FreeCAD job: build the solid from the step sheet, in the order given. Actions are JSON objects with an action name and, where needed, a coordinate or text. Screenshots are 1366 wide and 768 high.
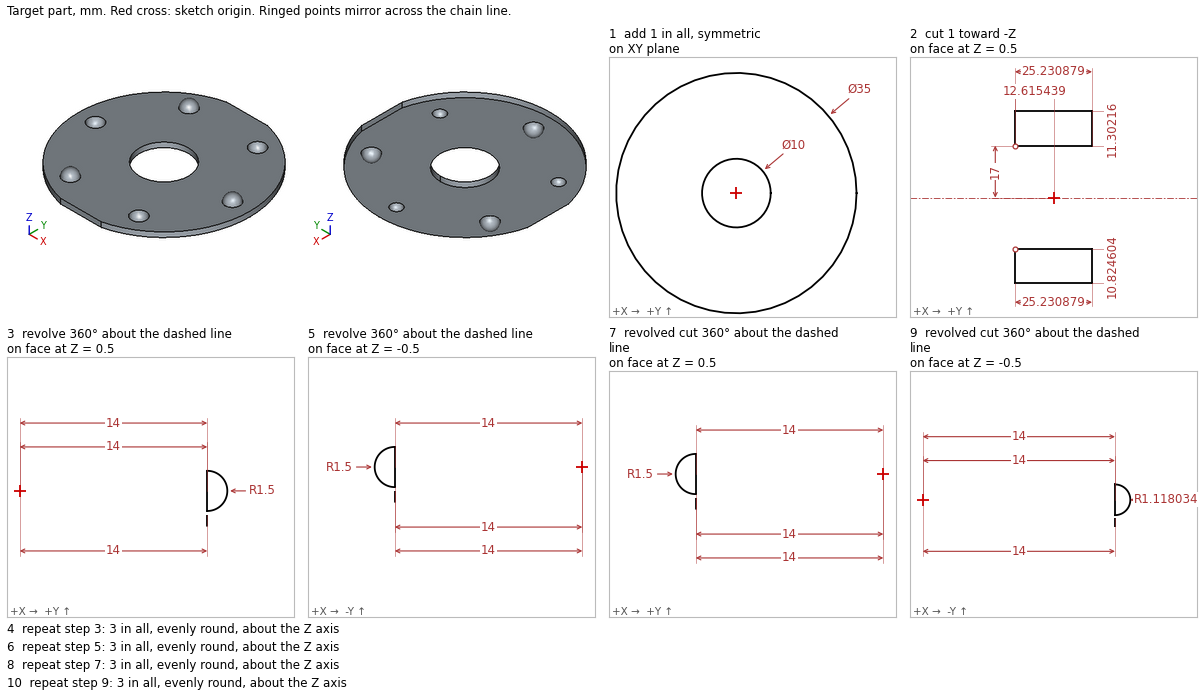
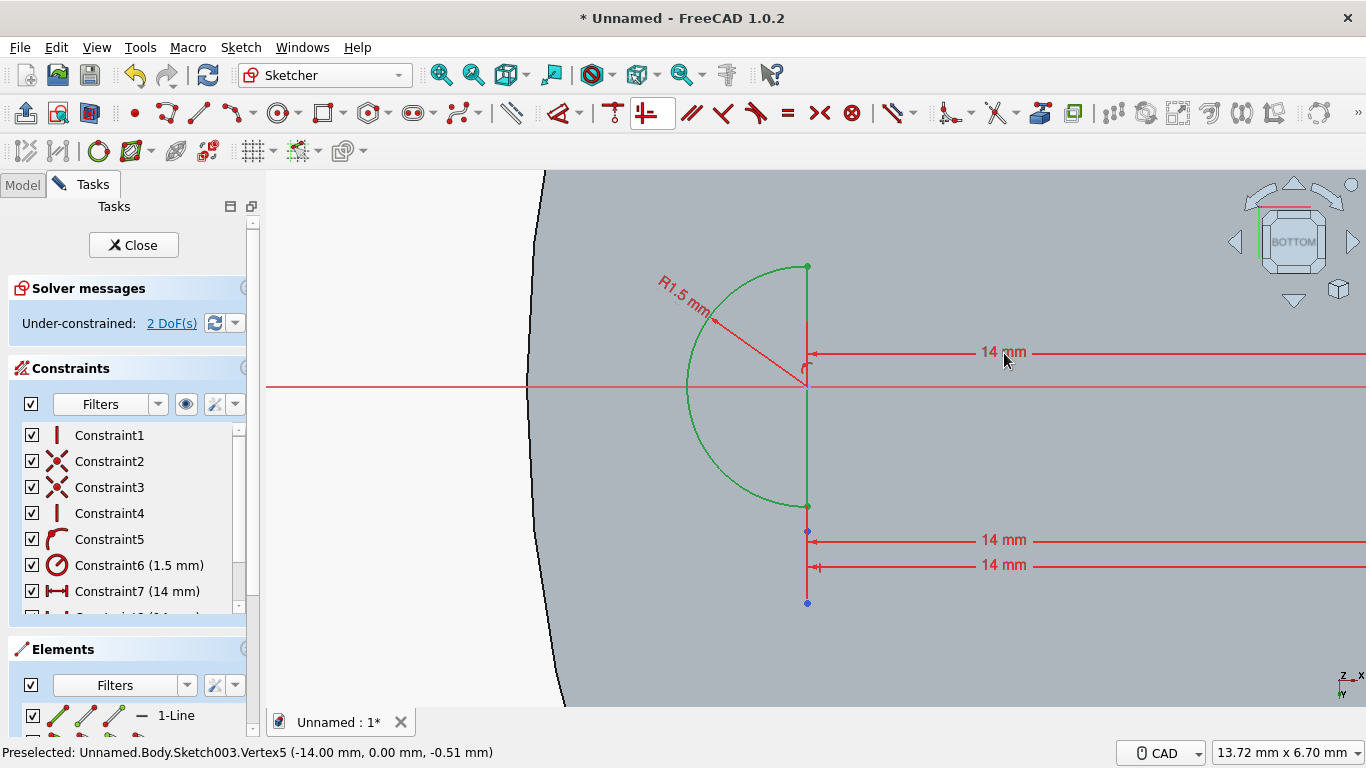
{"action": "left_click", "coordinate": [134, 245]}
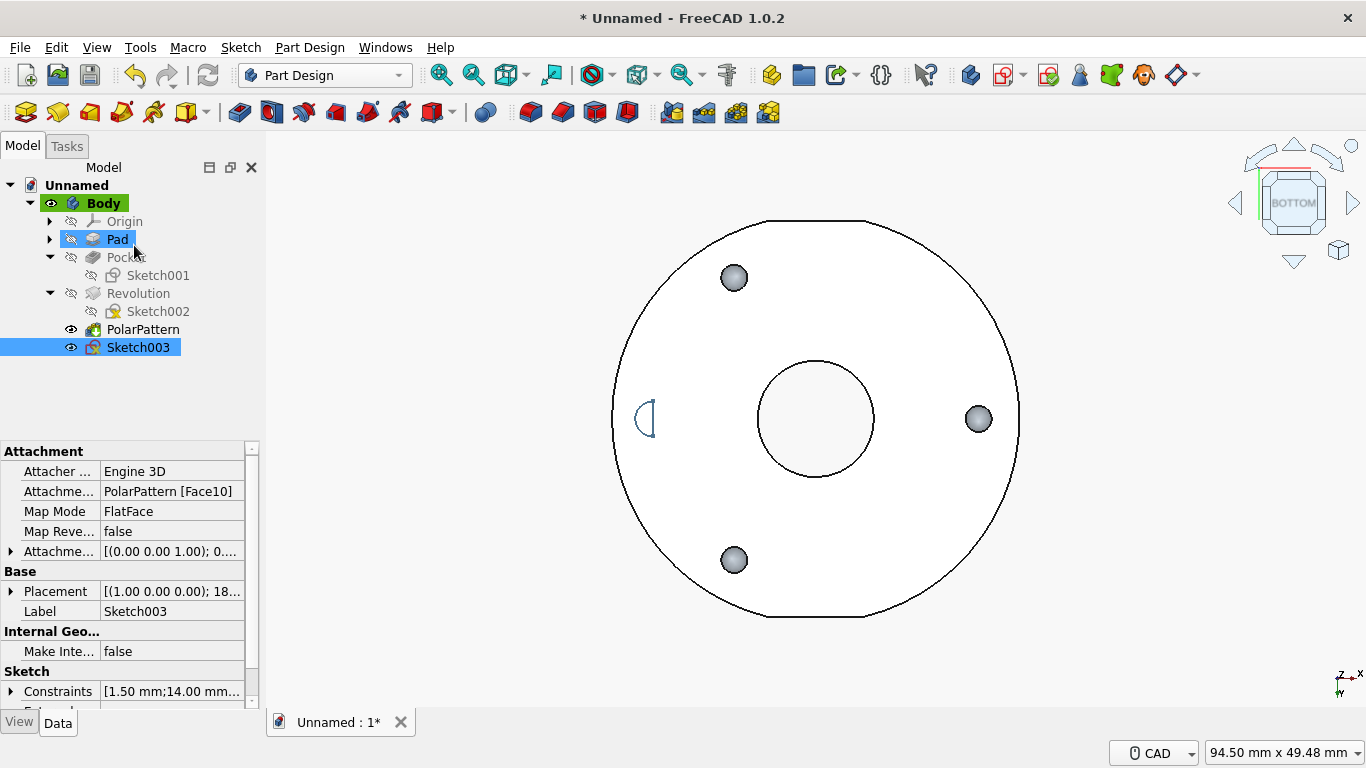
{"action": "left_click", "coordinate": [58, 112]}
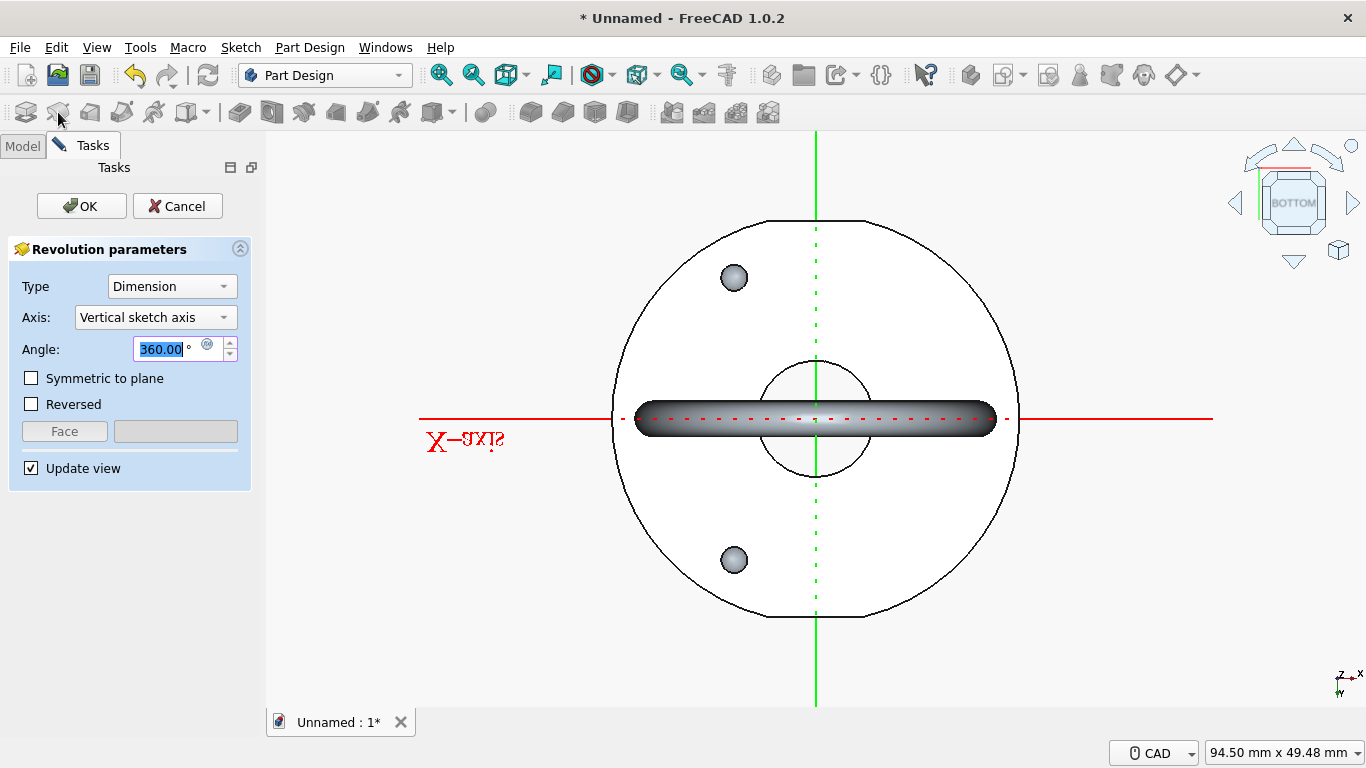
{"action": "left_click", "coordinate": [156, 318]}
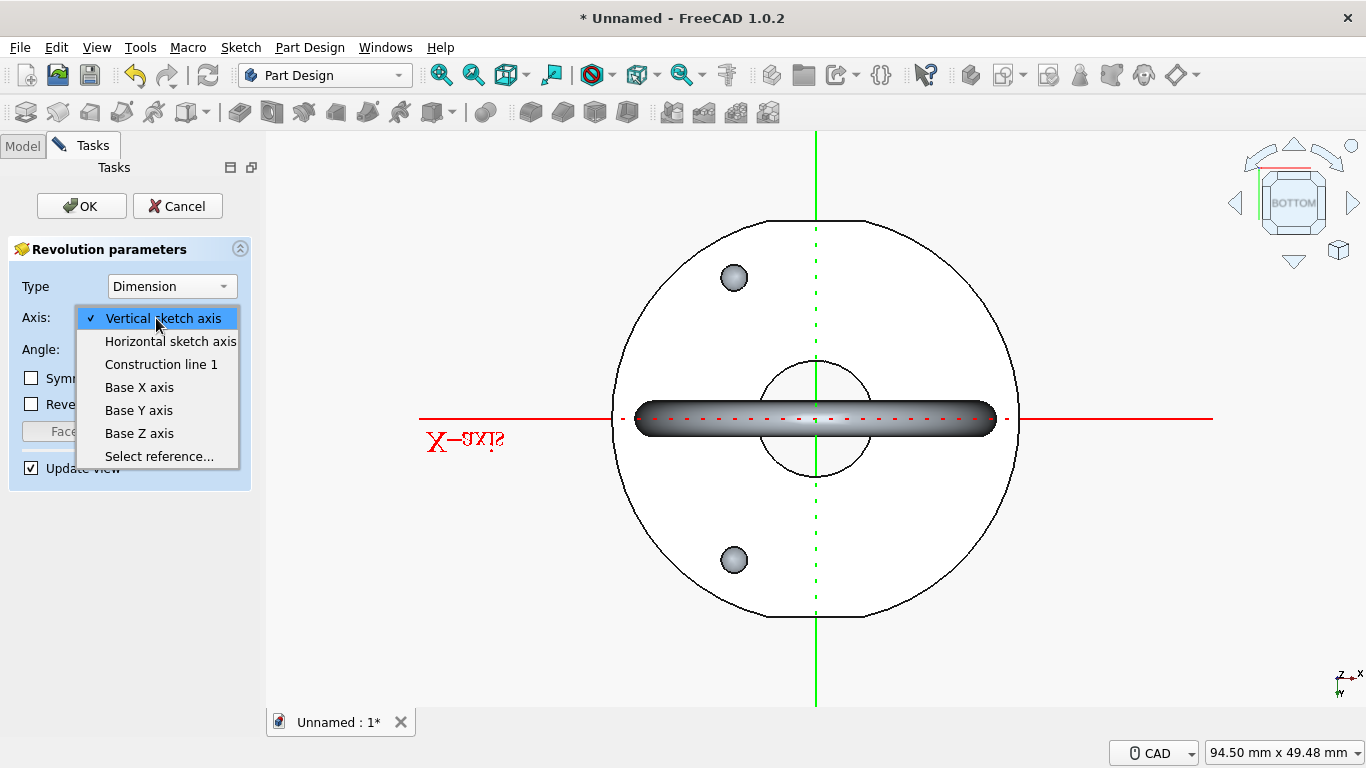
{"action": "left_click", "coordinate": [156, 364]}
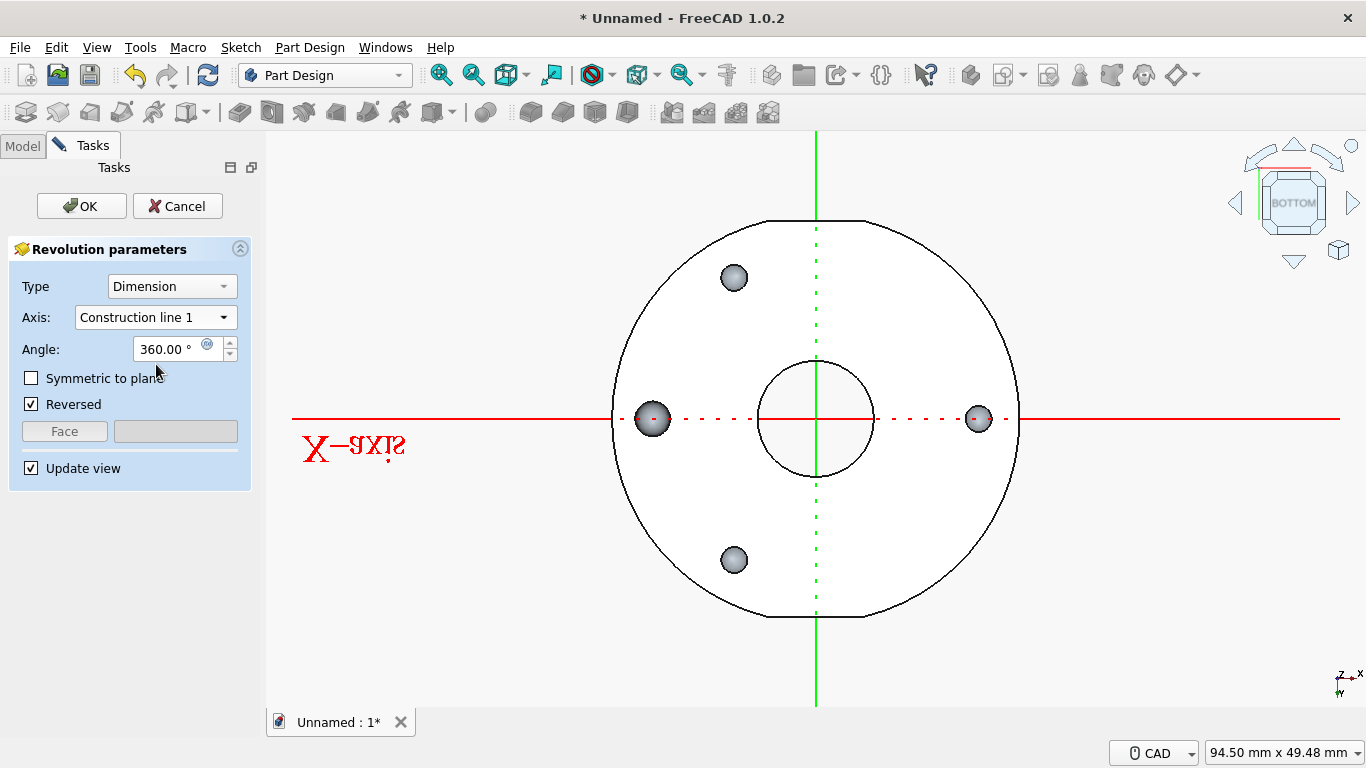
{"action": "left_click", "coordinate": [82, 206]}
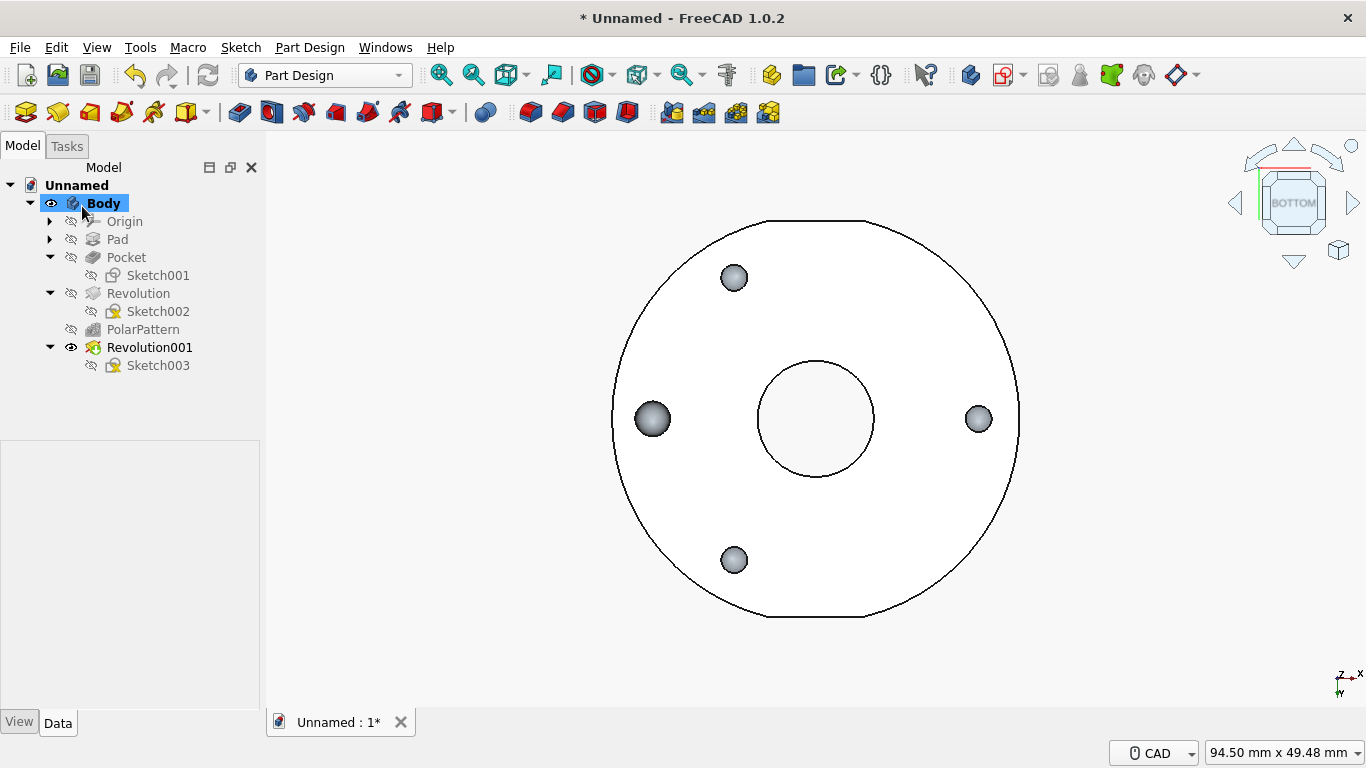
{"action": "left_click", "coordinate": [116, 347]}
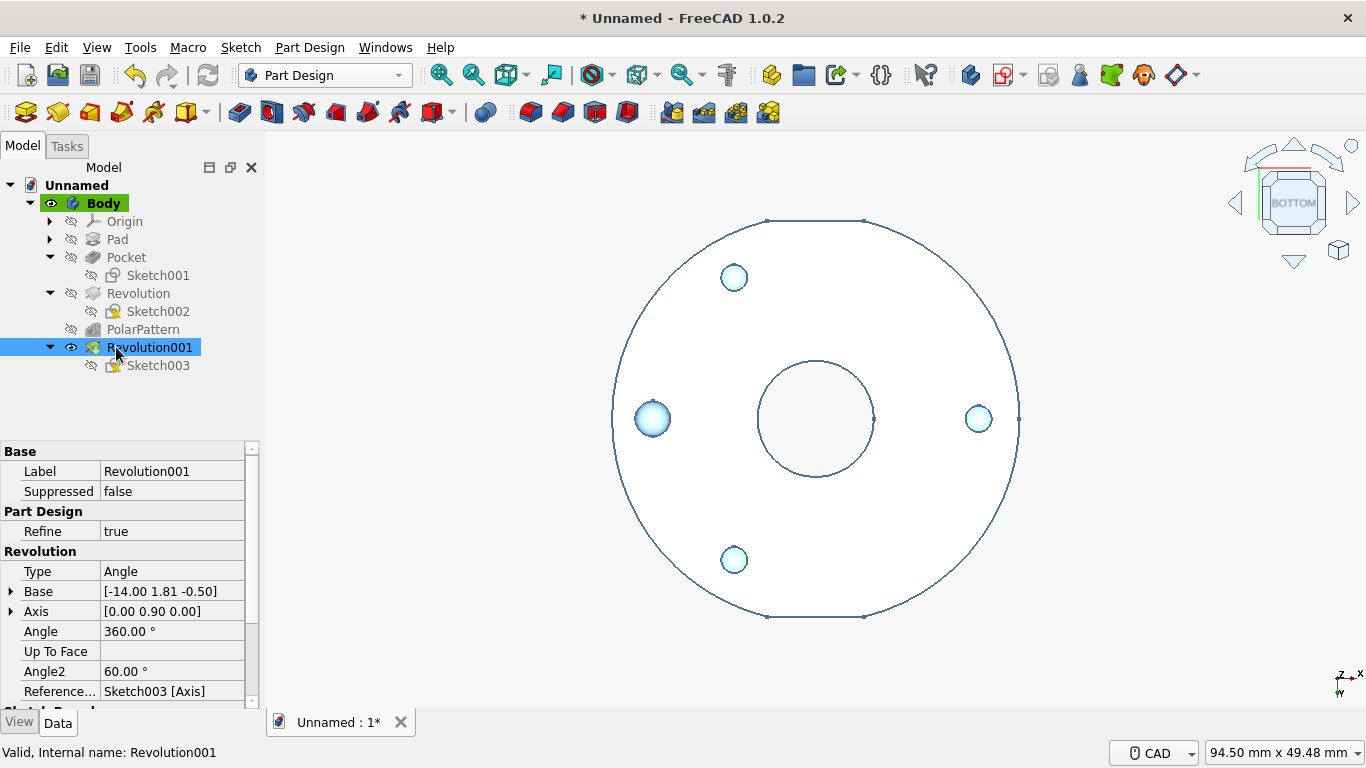
{"action": "left_click", "coordinate": [736, 112]}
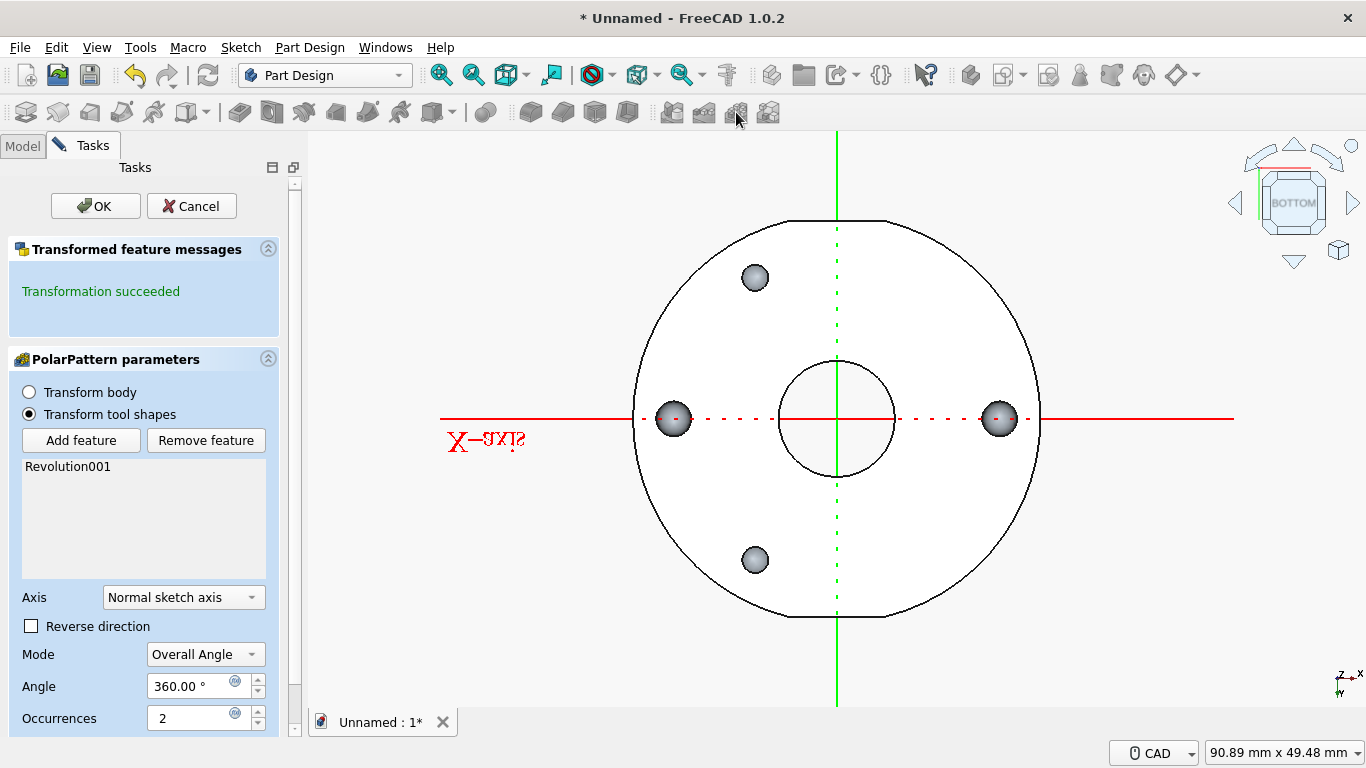
{"action": "left_click", "coordinate": [184, 598]}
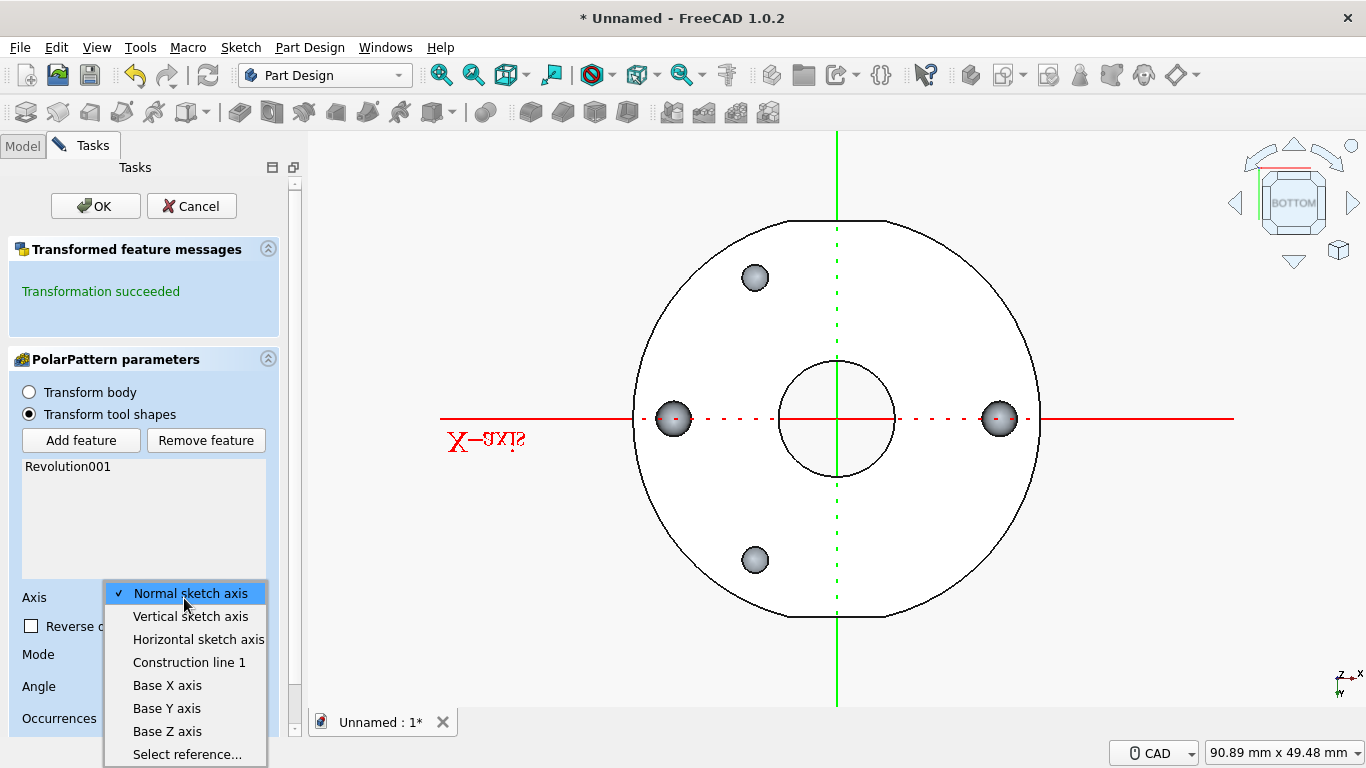
{"action": "left_click", "coordinate": [184, 732]}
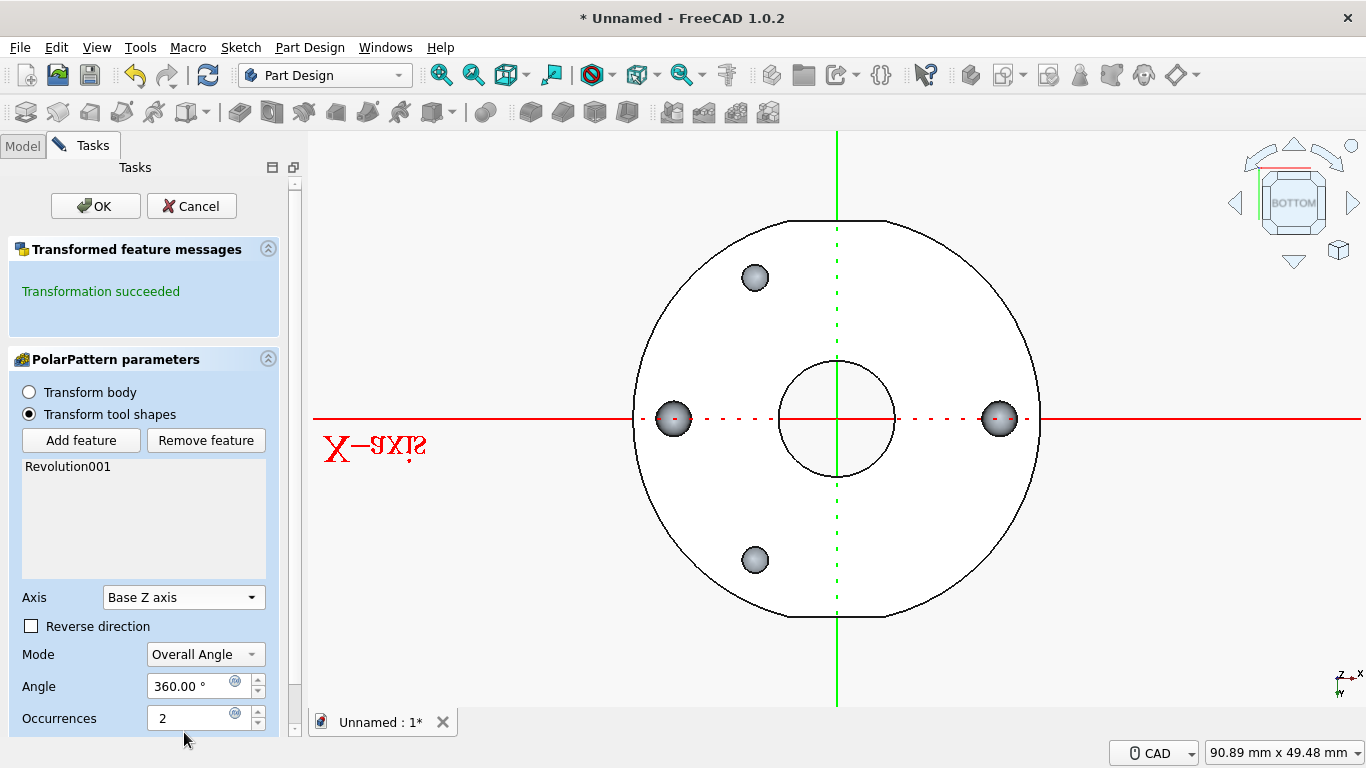
{"action": "triple_click", "coordinate": [198, 718]}